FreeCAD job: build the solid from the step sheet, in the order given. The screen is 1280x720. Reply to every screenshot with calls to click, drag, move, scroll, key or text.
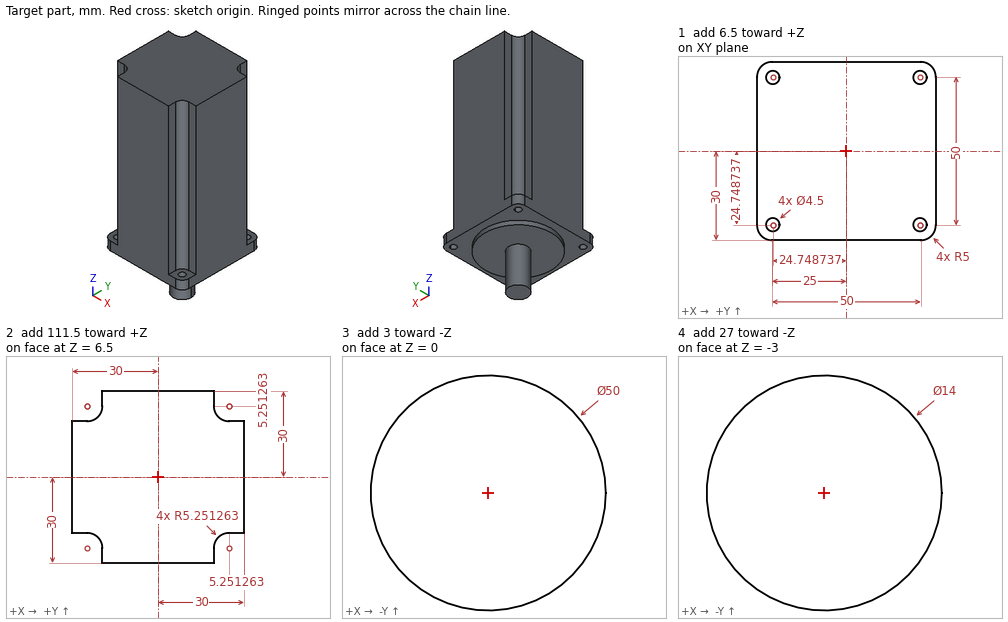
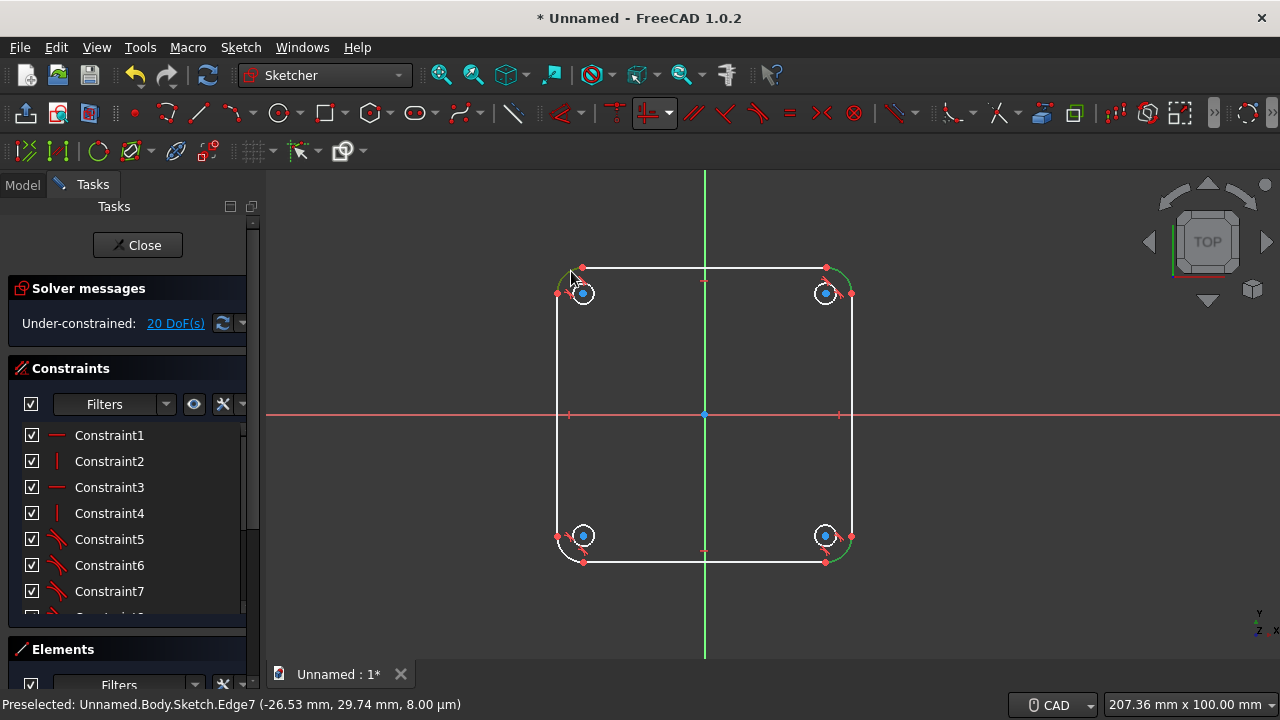
click(560, 548)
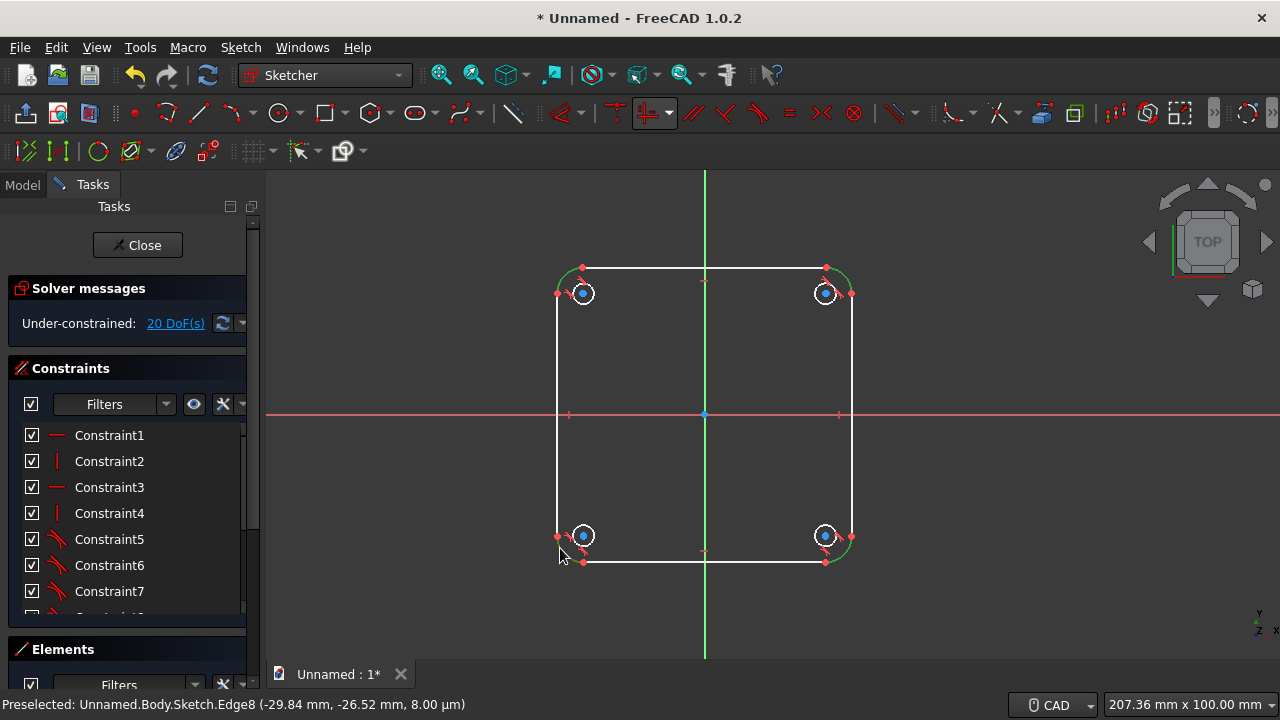
click(790, 114)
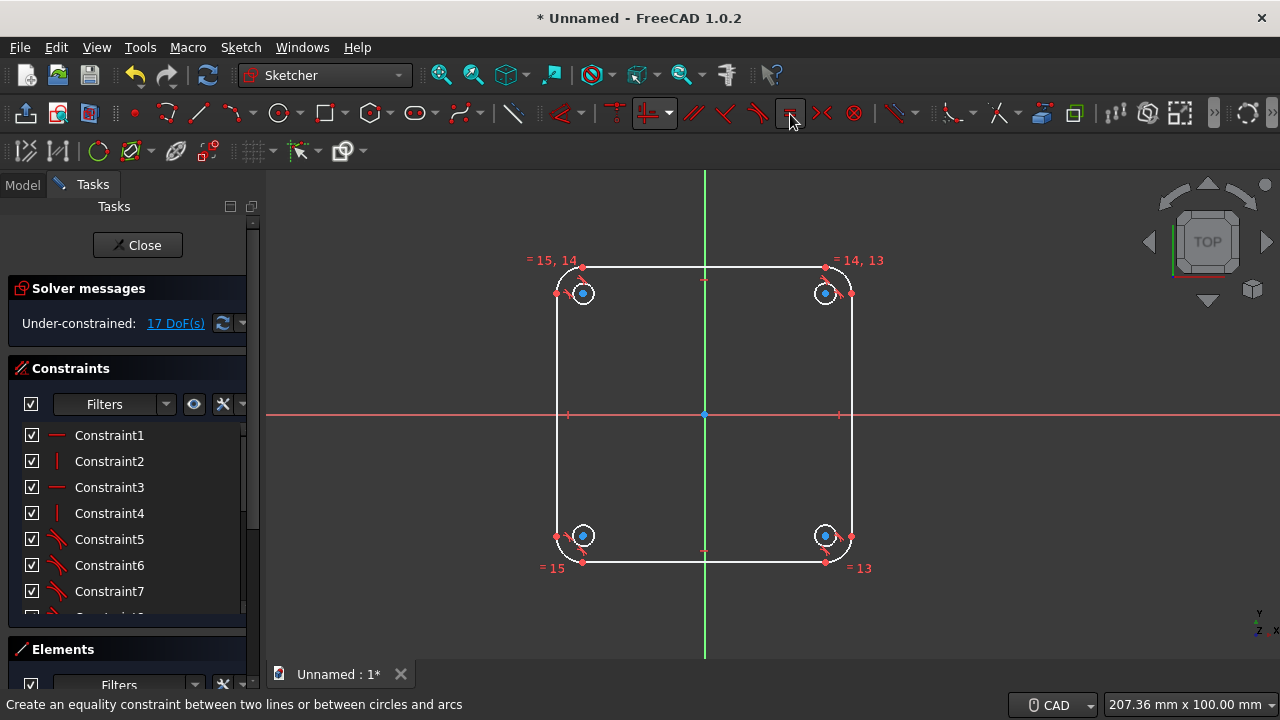
scroll(591, 528, up, 2)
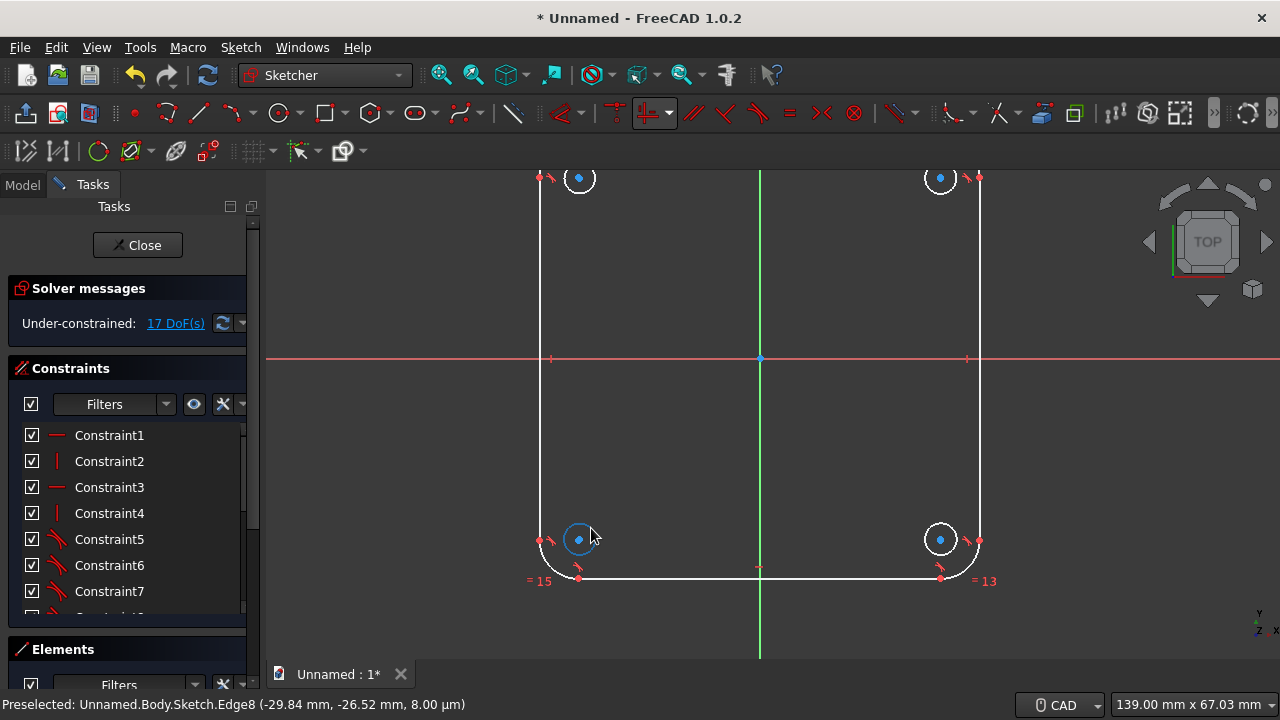
click(591, 528)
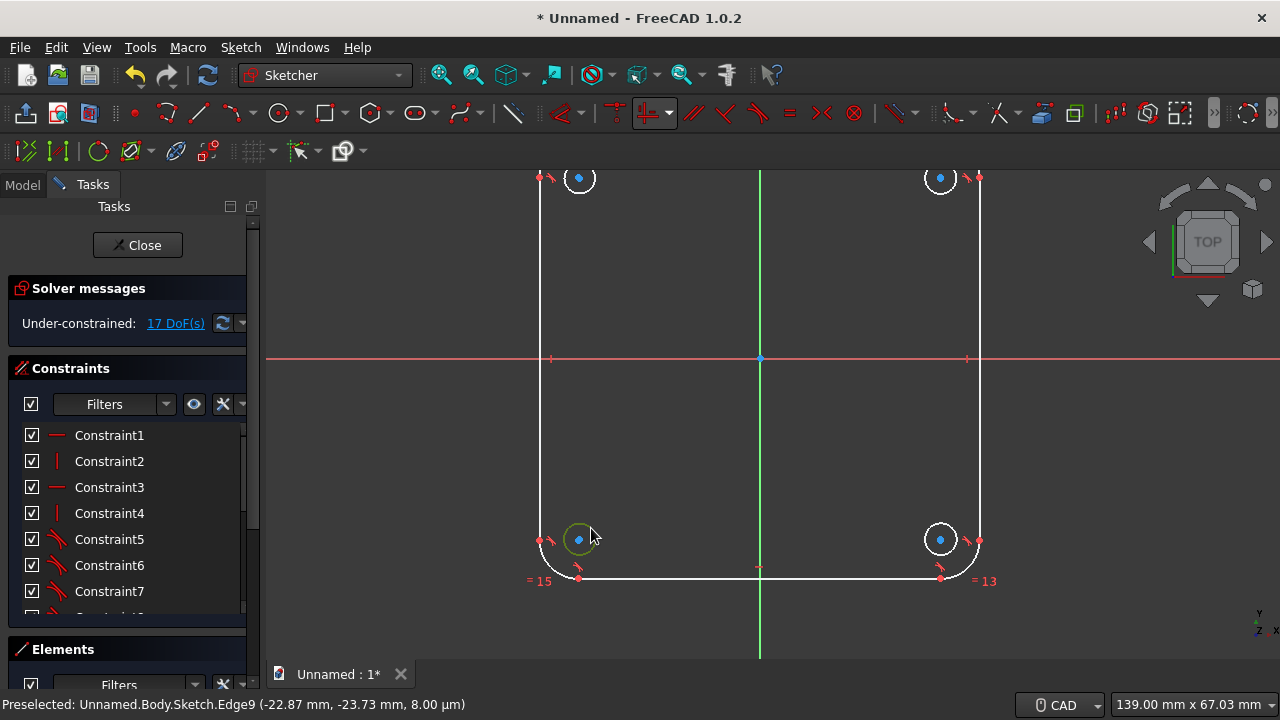
click(952, 528)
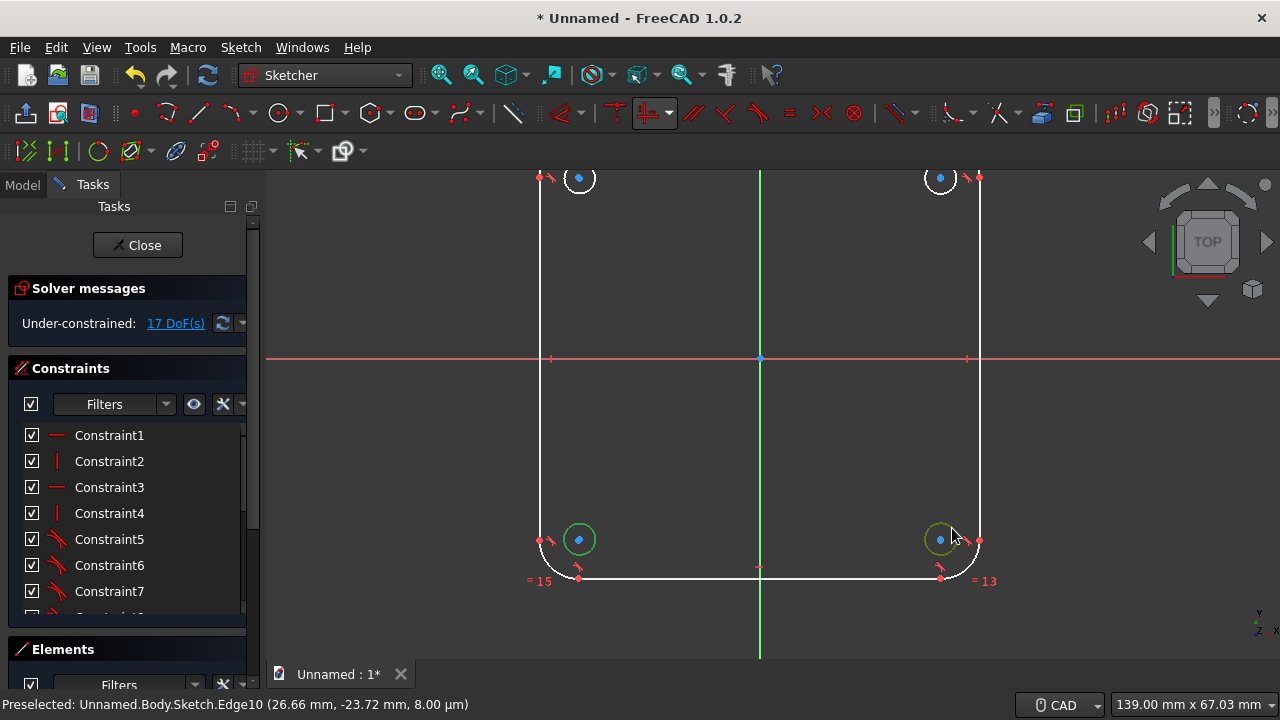
scroll(591, 528, down, 2)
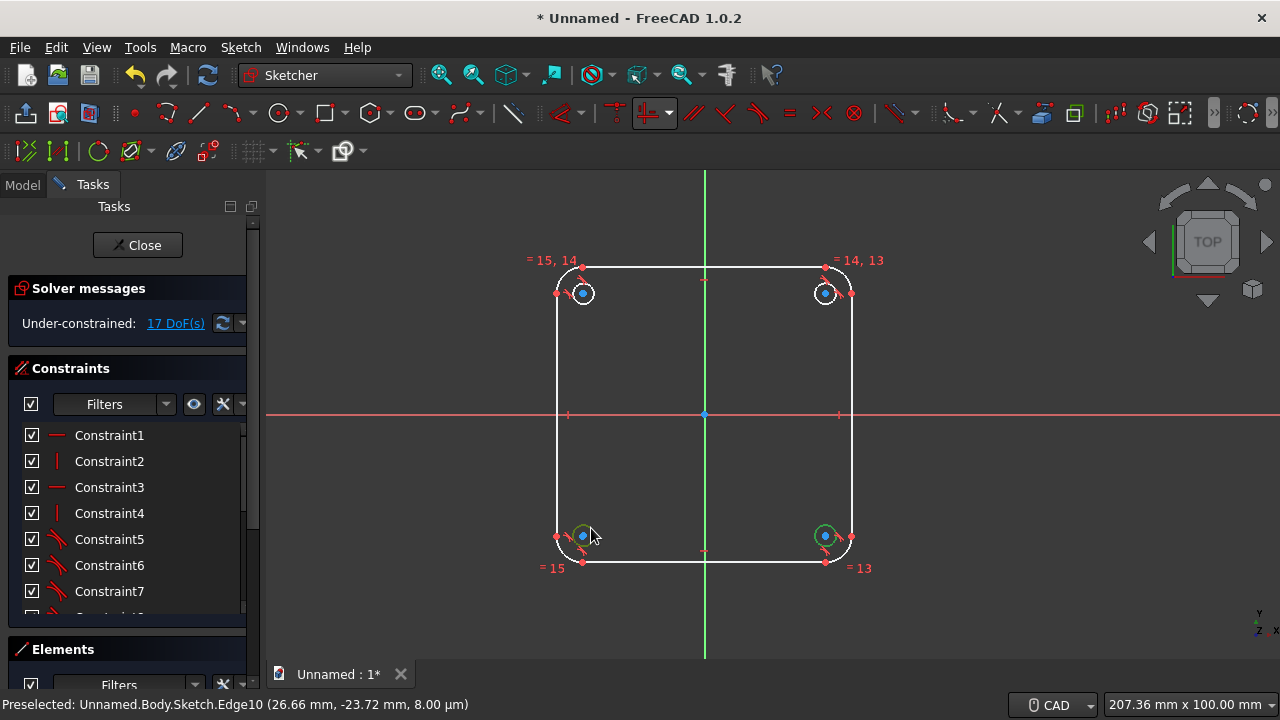
scroll(591, 286, up, 2)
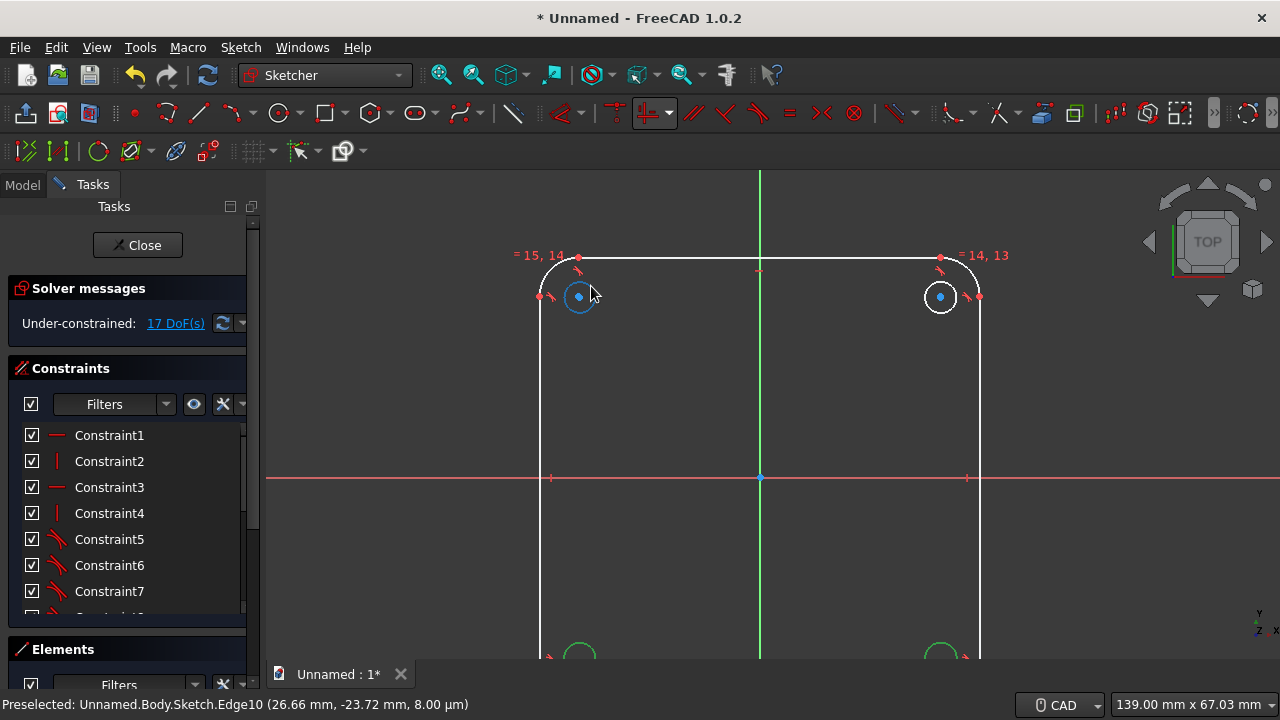
click(591, 287)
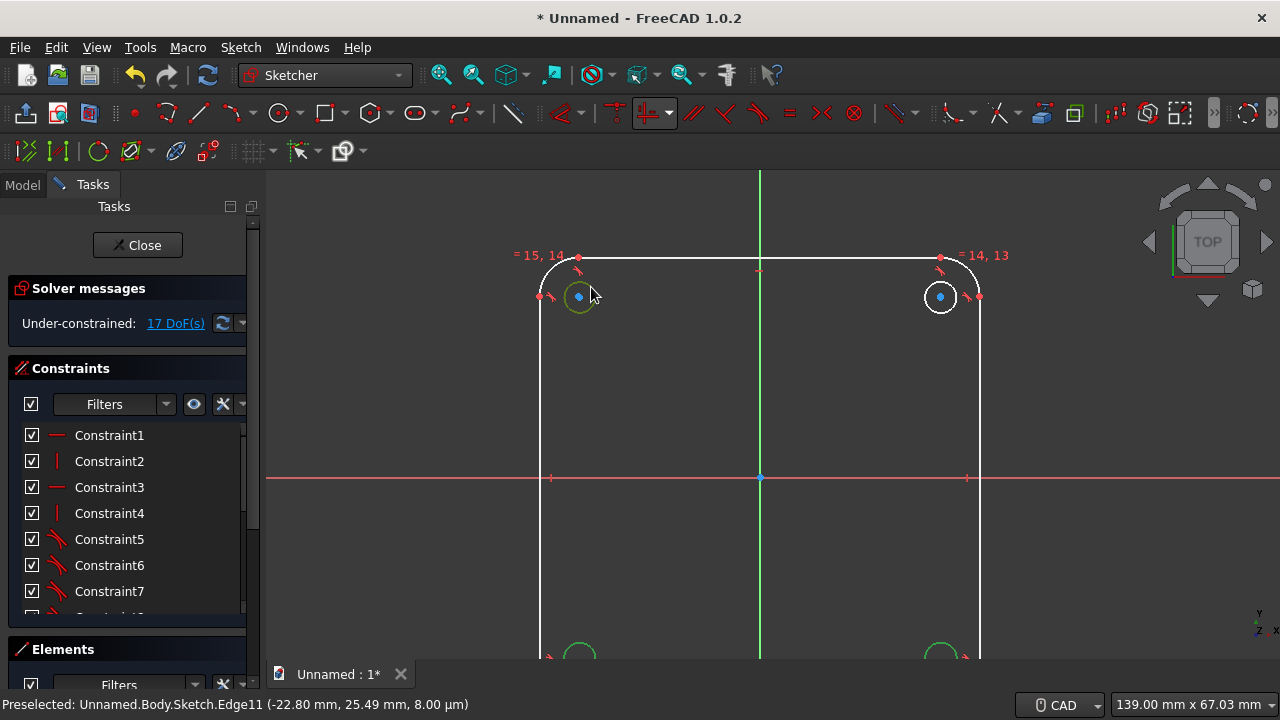
click(952, 286)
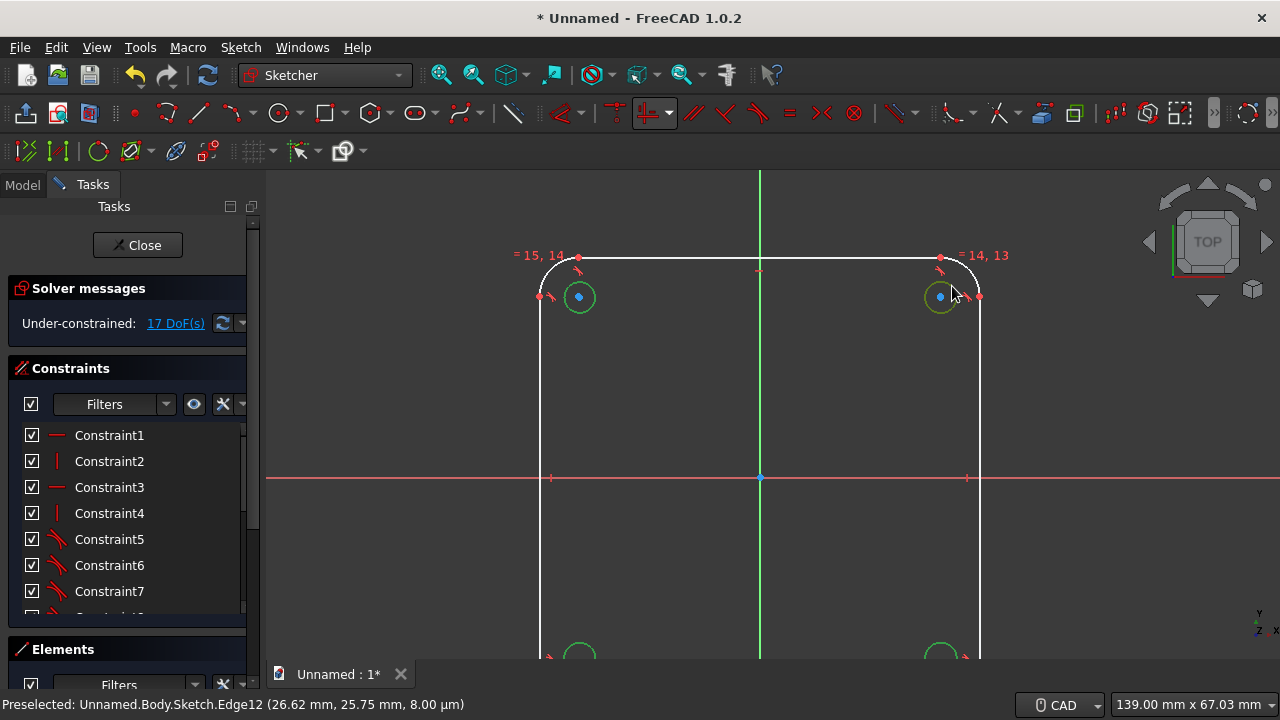
click(790, 114)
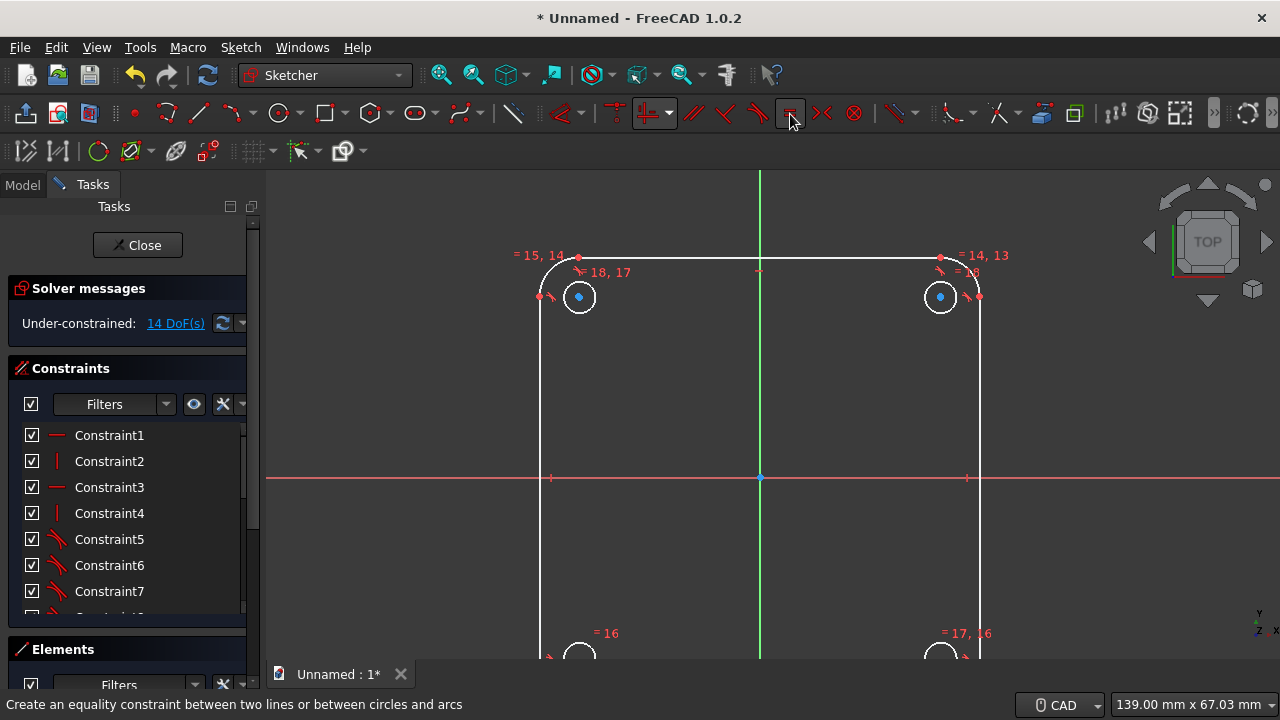
scroll(591, 286, down, 2)